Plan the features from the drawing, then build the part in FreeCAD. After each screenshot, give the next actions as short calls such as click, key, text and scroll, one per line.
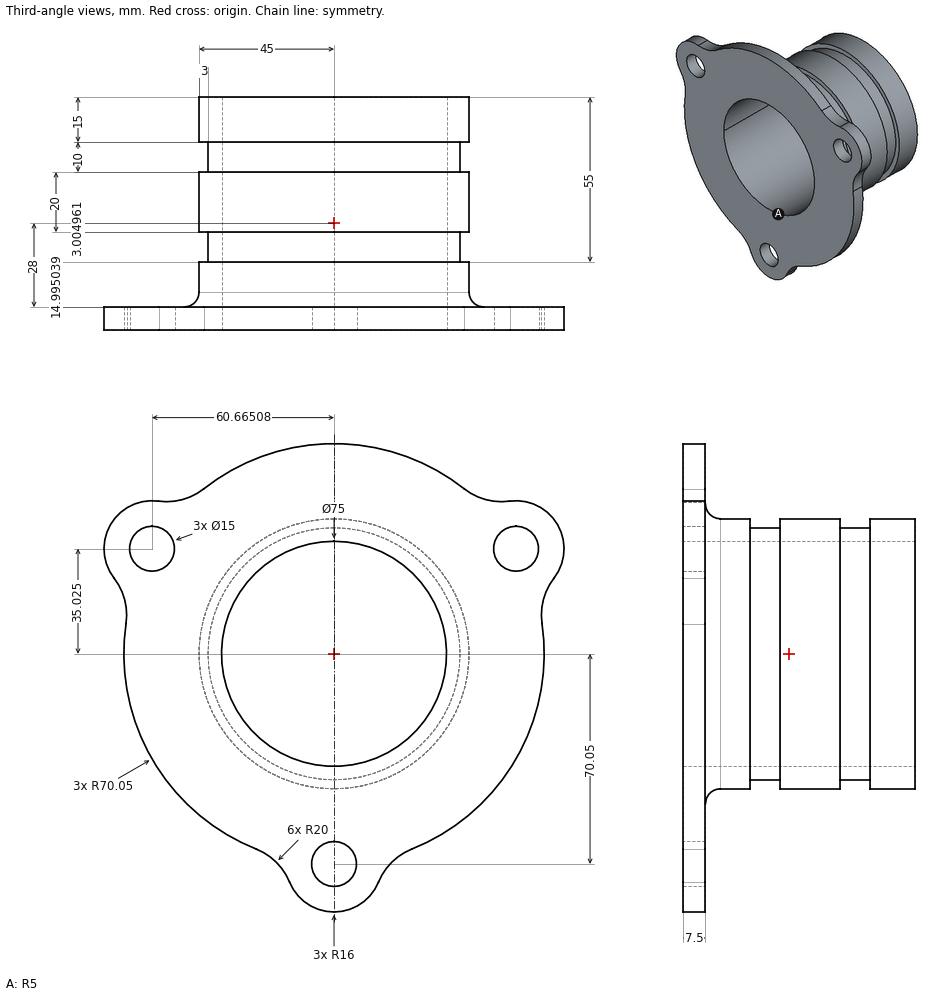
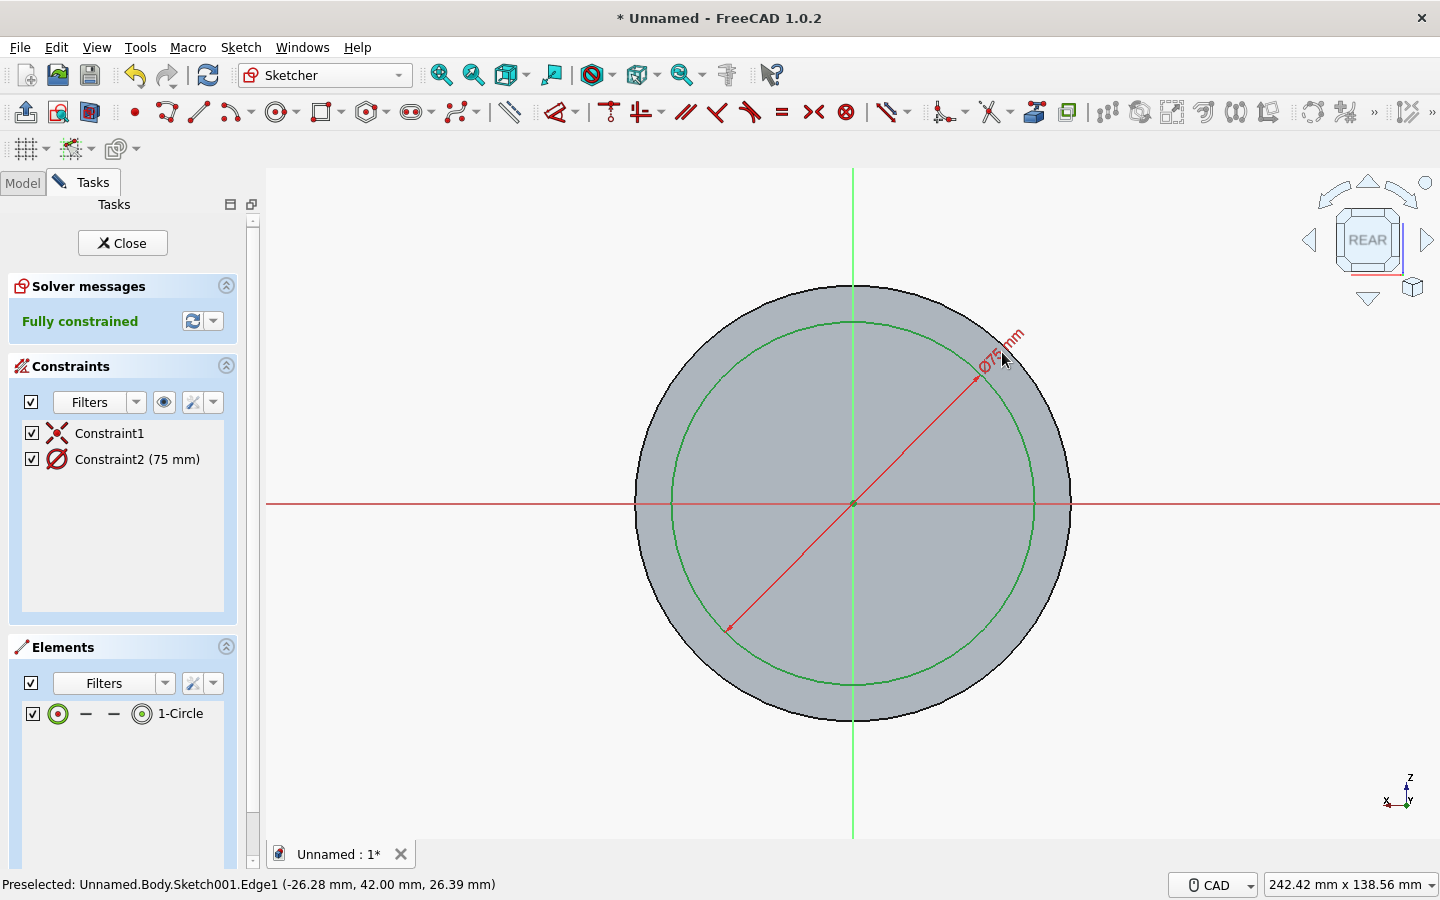
click(123, 243)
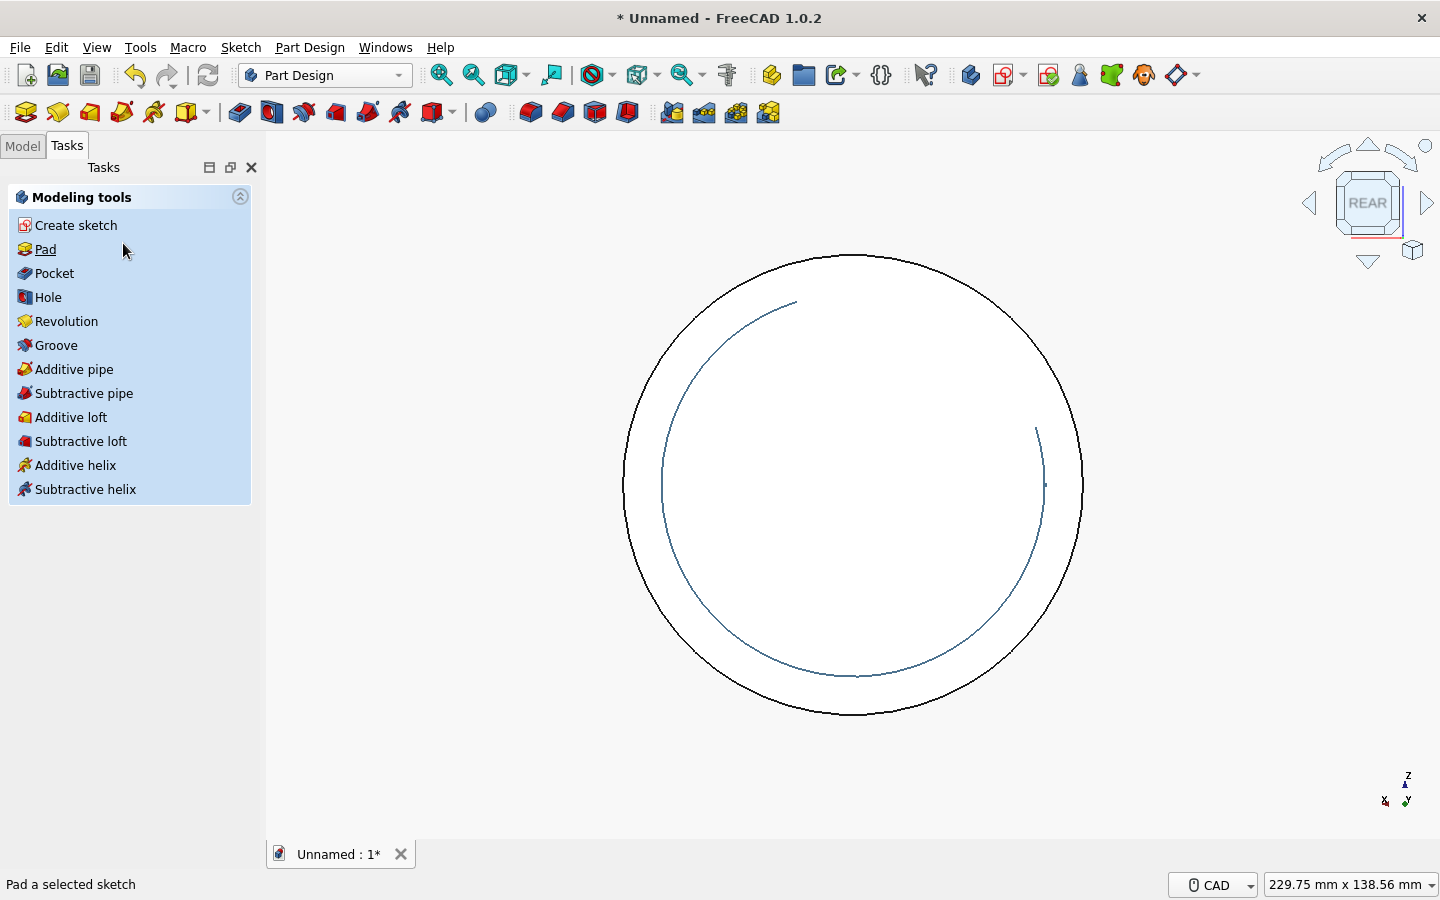
click(240, 112)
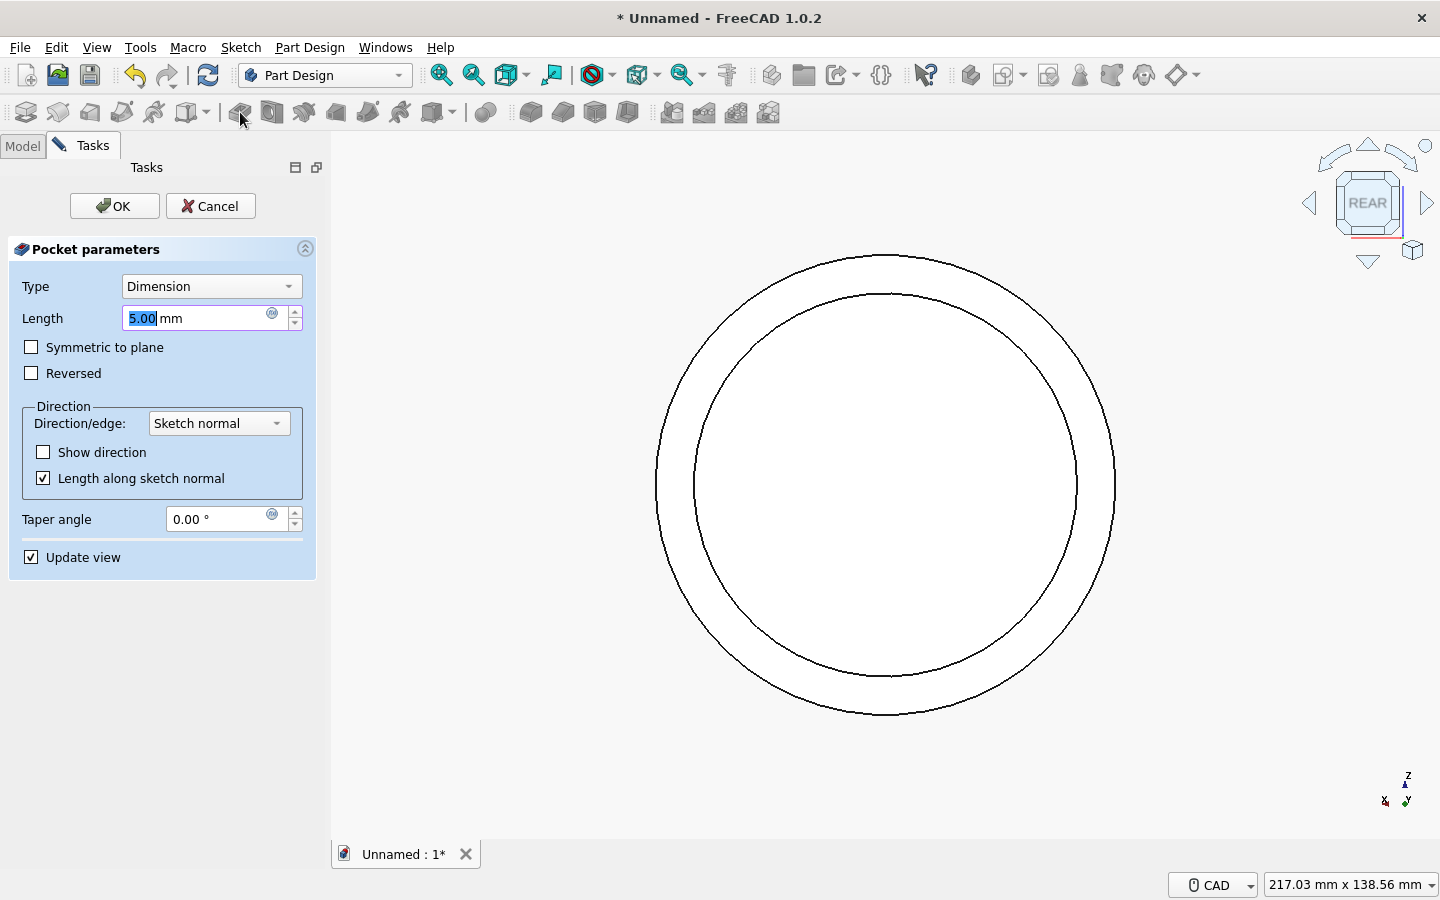
click(212, 286)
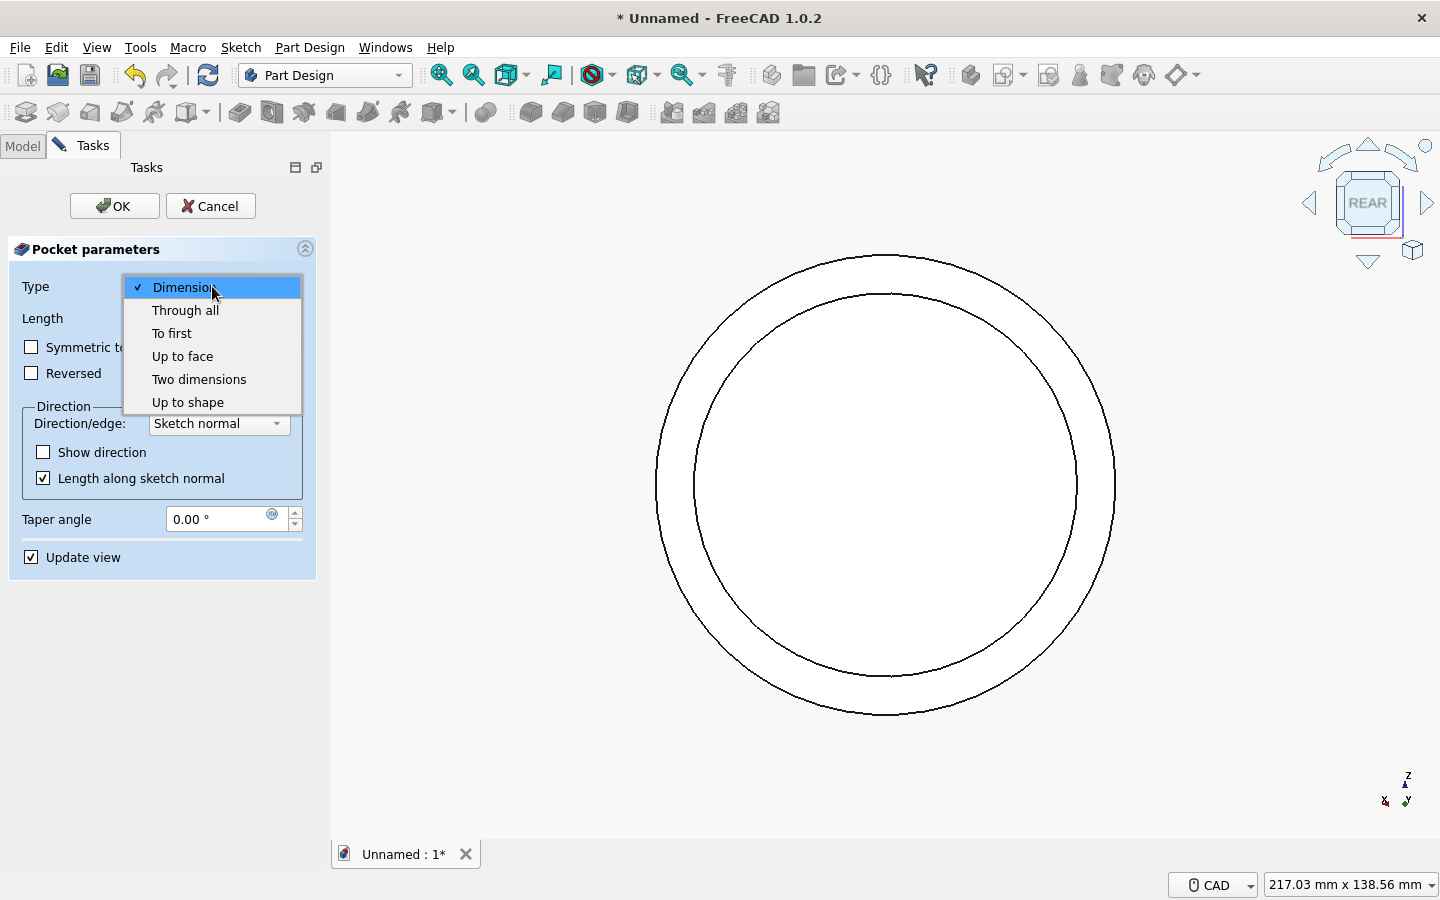
click(212, 310)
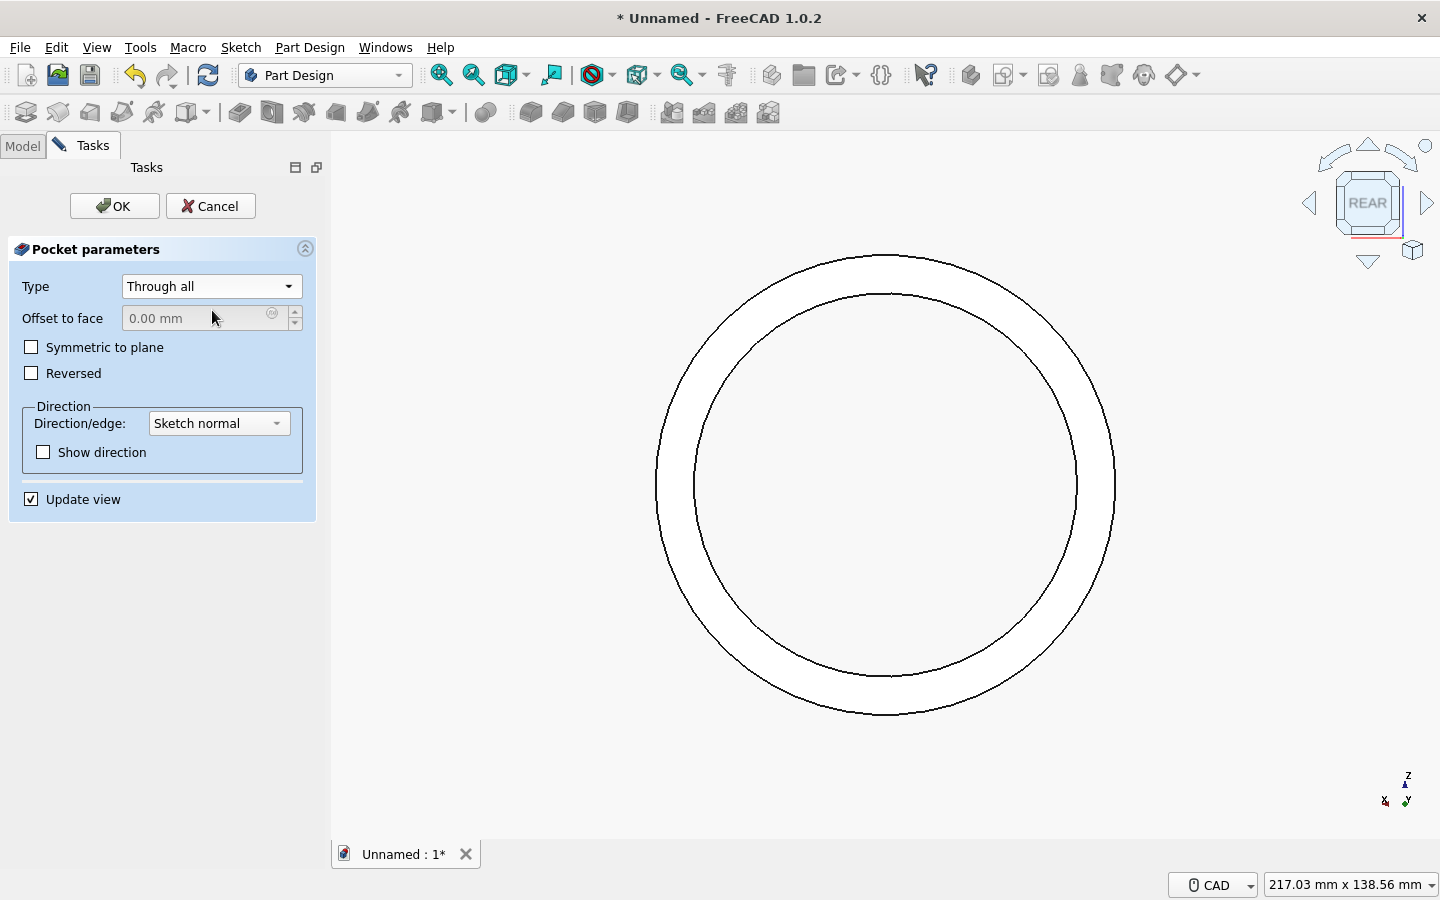
click(115, 206)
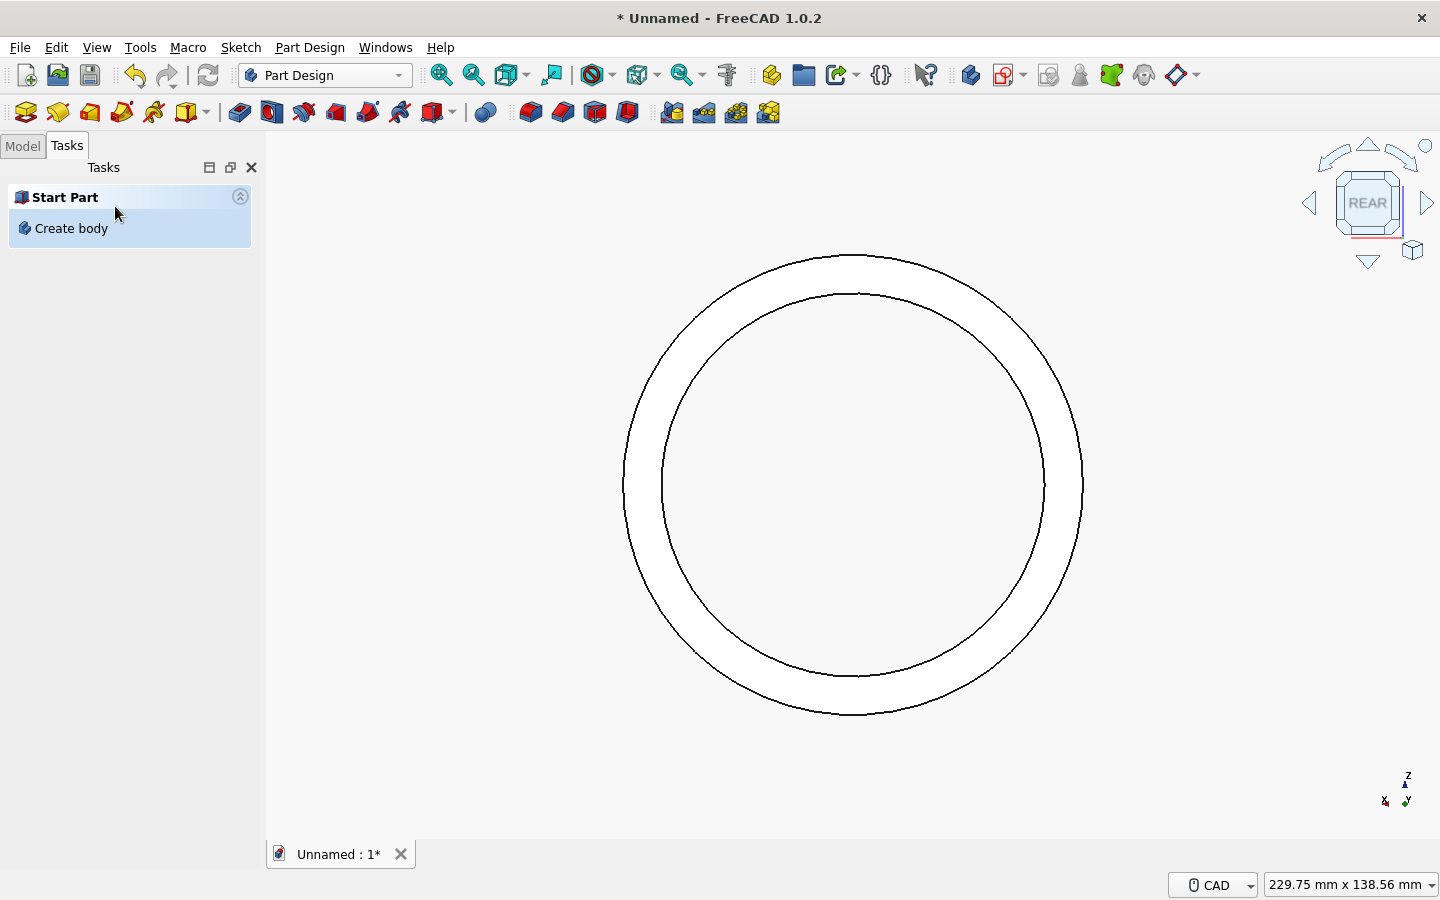
click(972, 76)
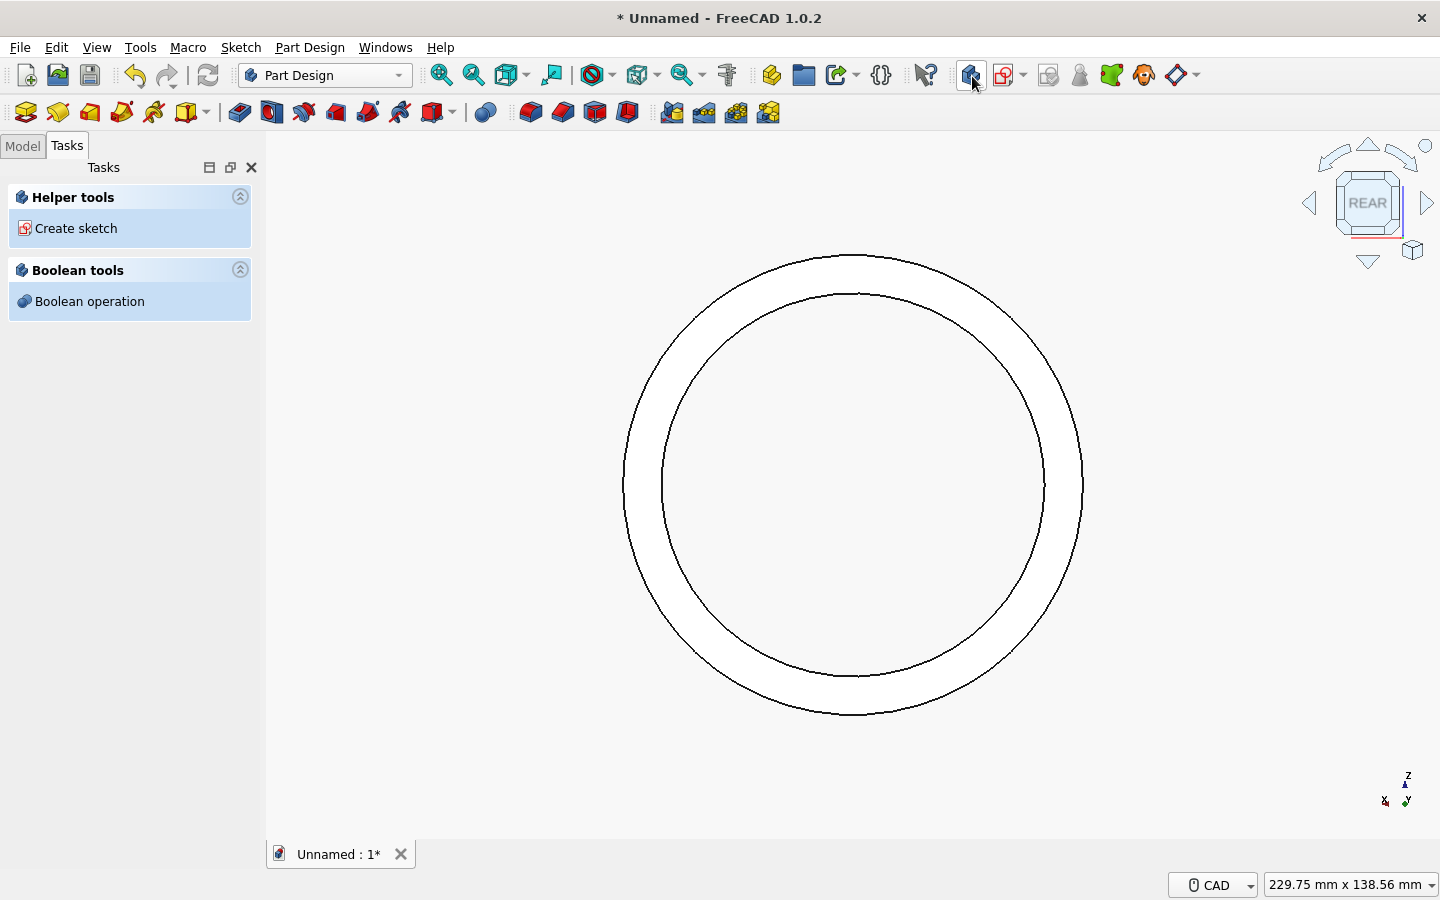
click(23, 145)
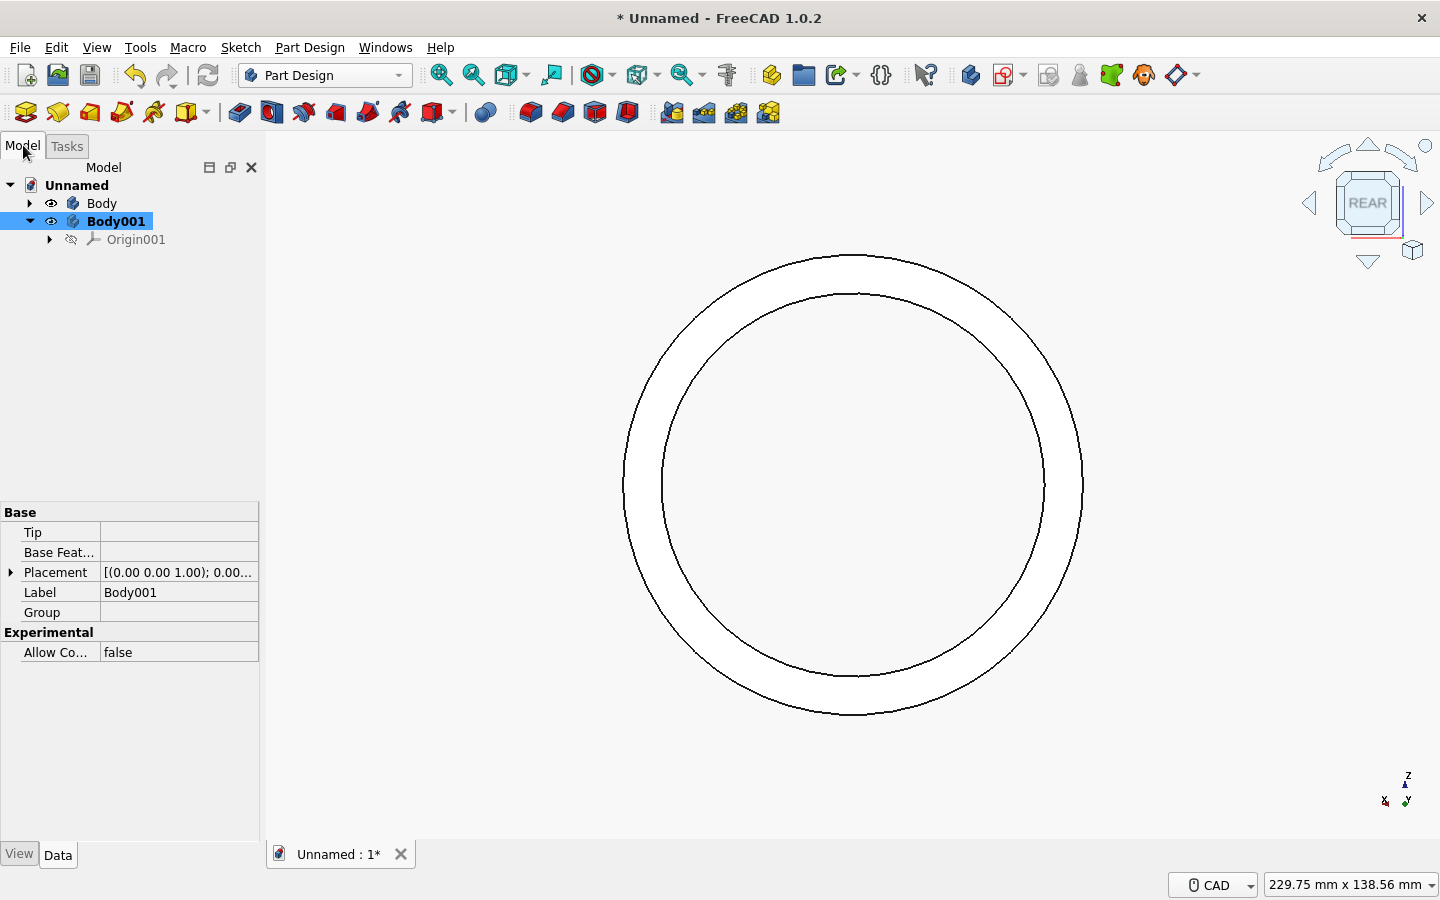
click(50, 239)